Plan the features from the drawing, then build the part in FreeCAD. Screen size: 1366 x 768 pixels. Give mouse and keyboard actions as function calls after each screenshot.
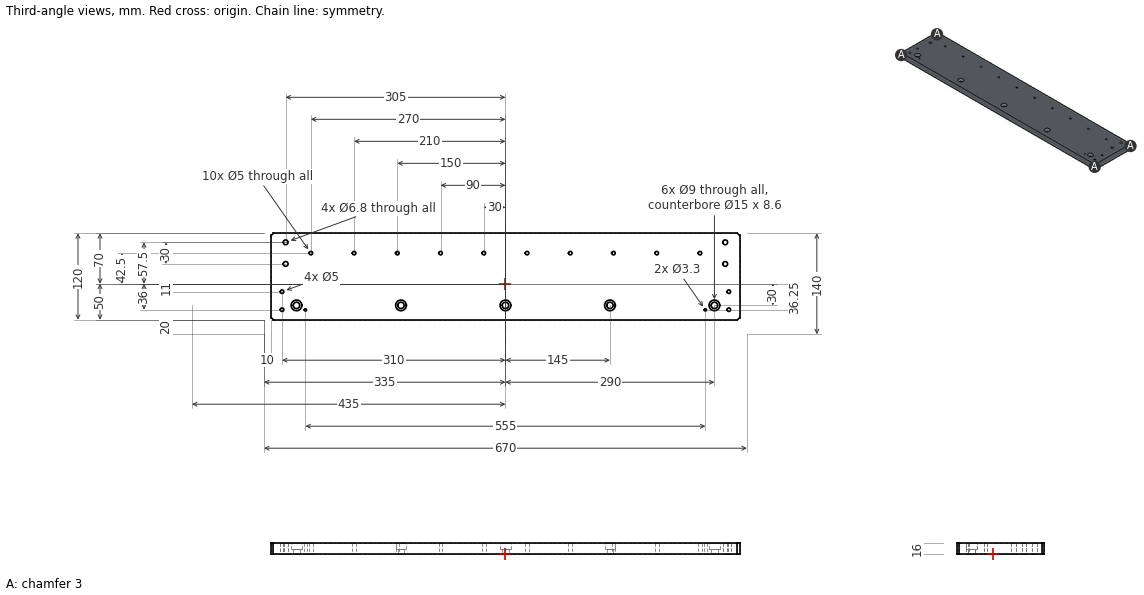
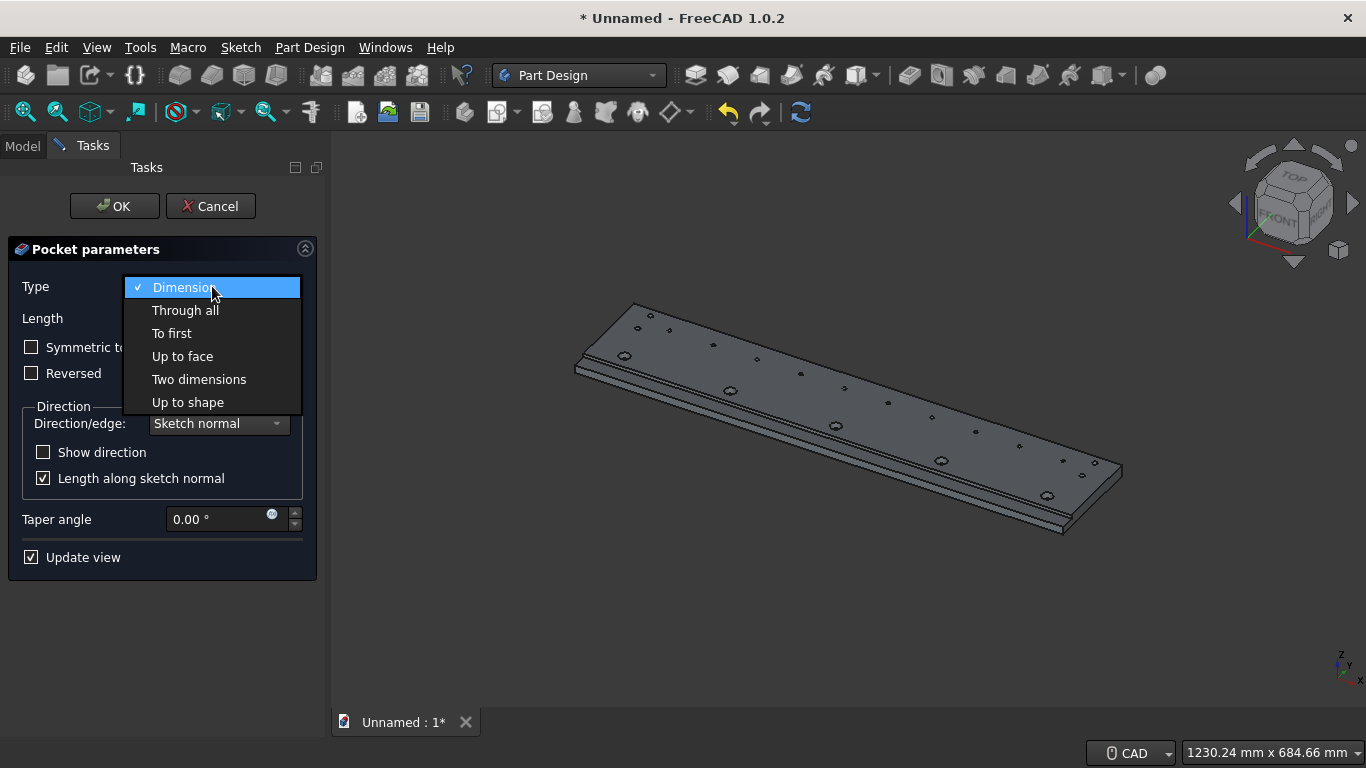
click(212, 310)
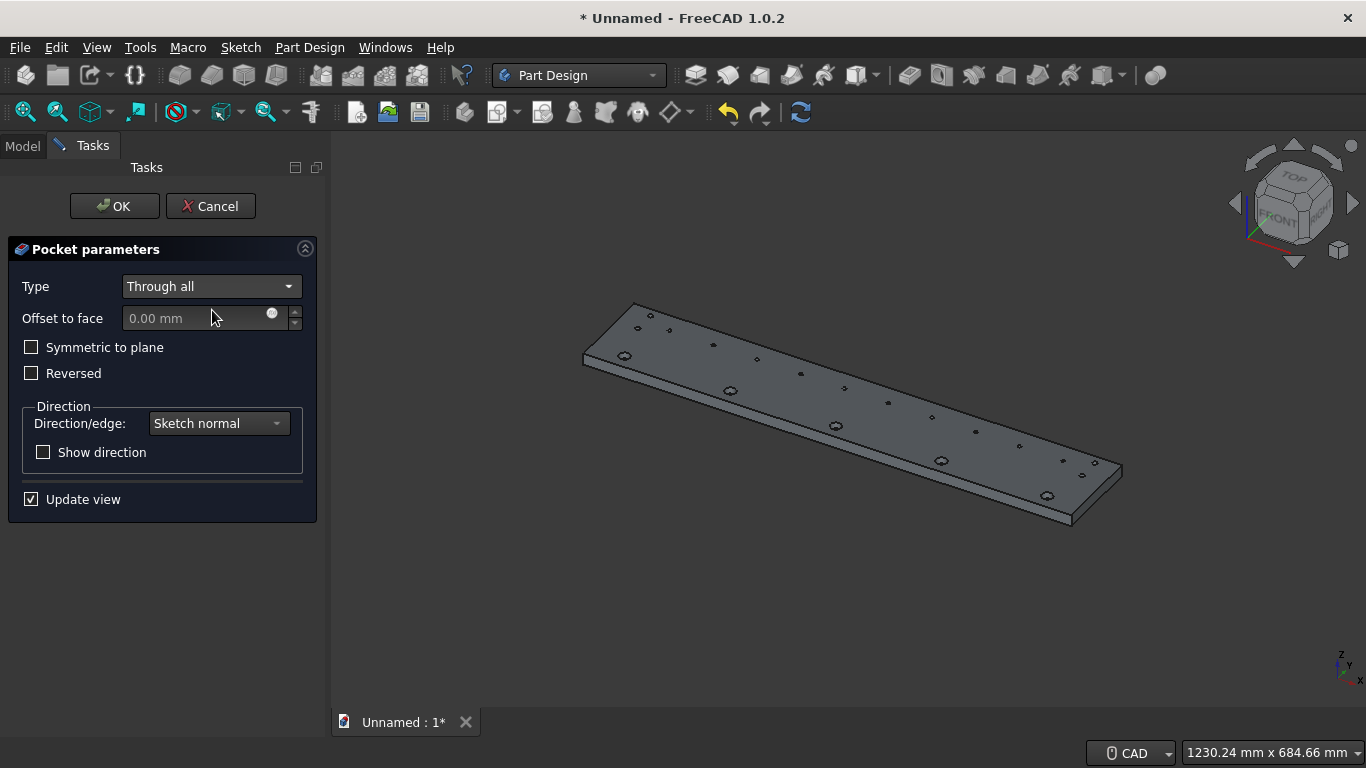
click(115, 206)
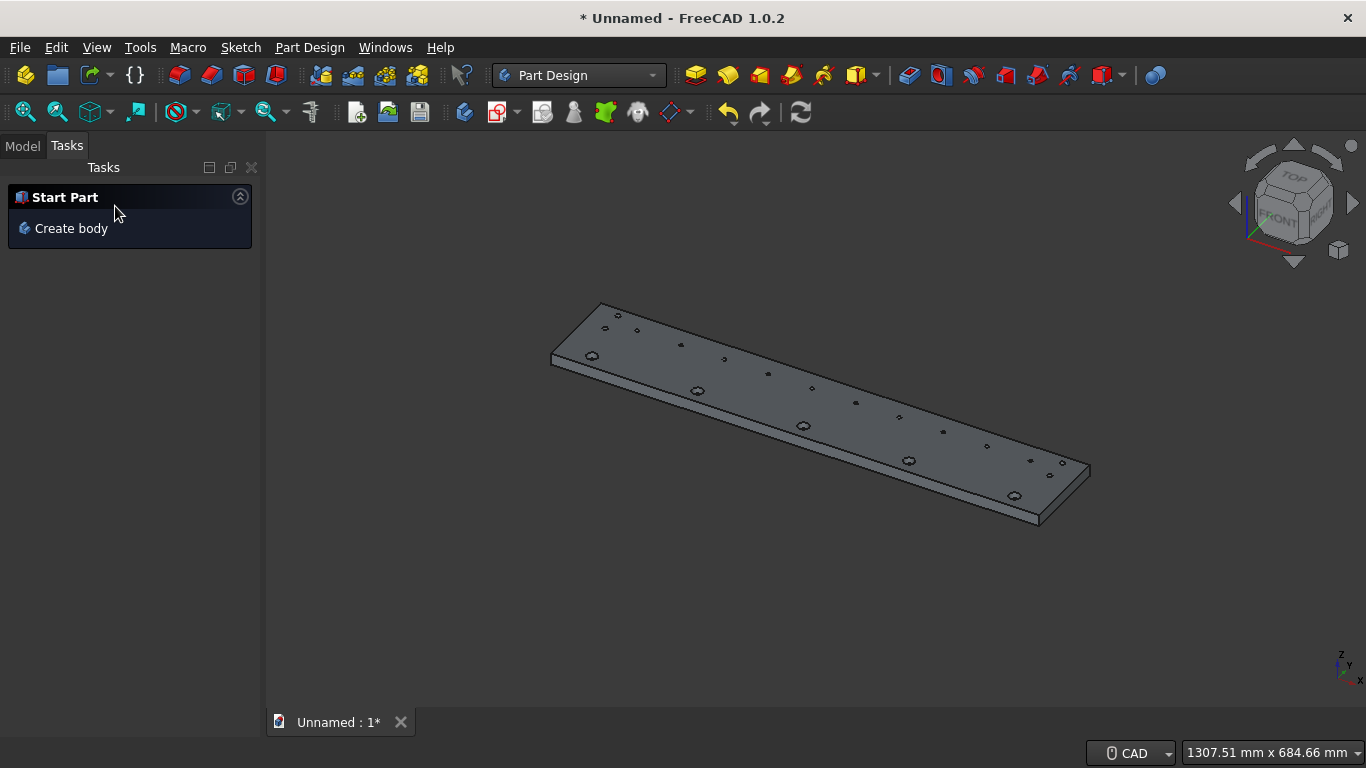
click(952, 462)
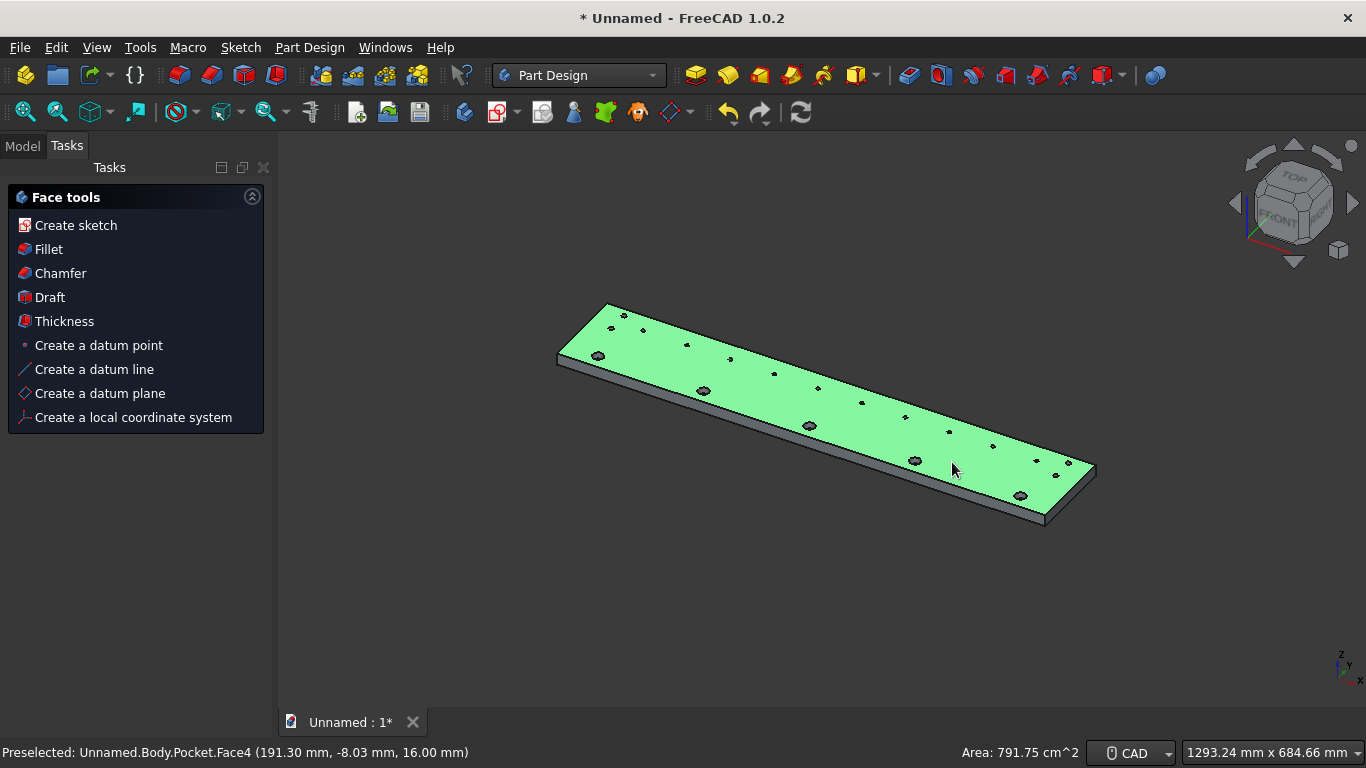
click(498, 112)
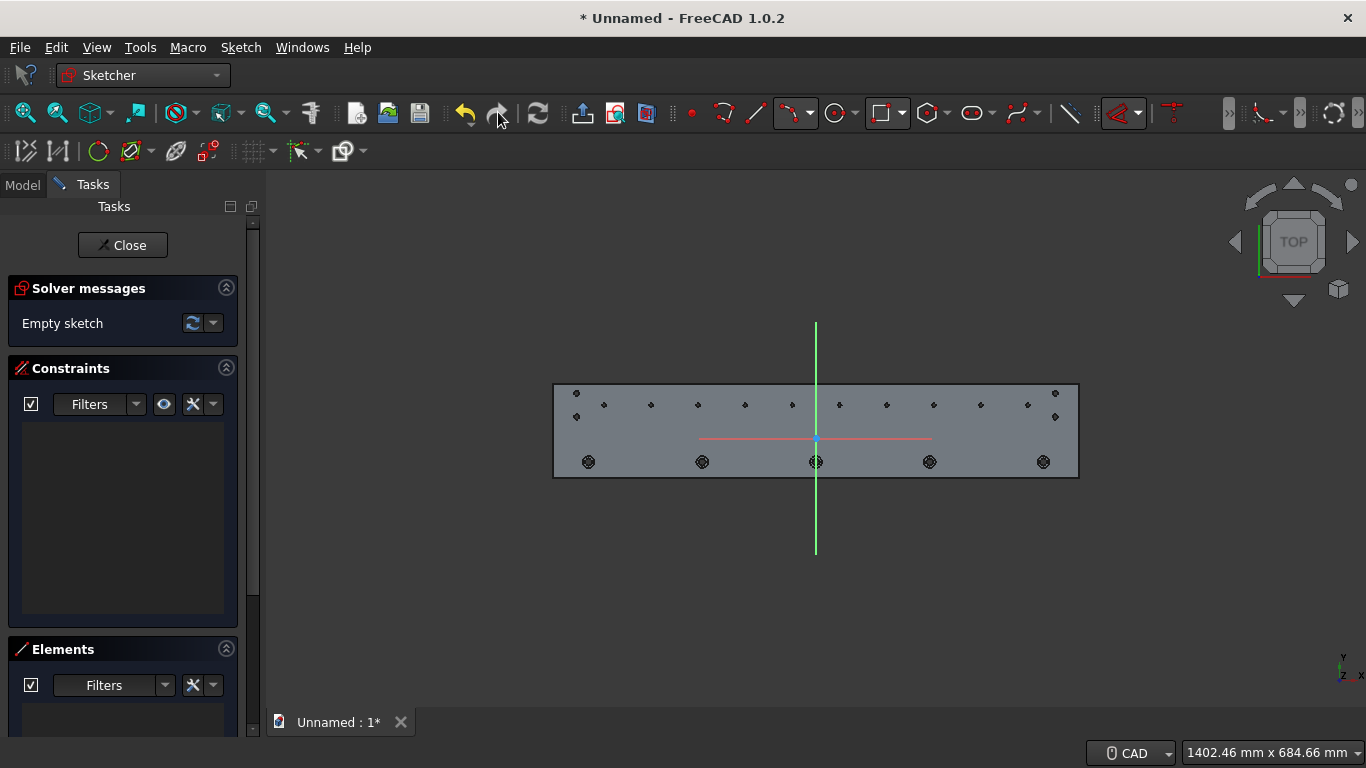
scroll(475, 427, up, 6)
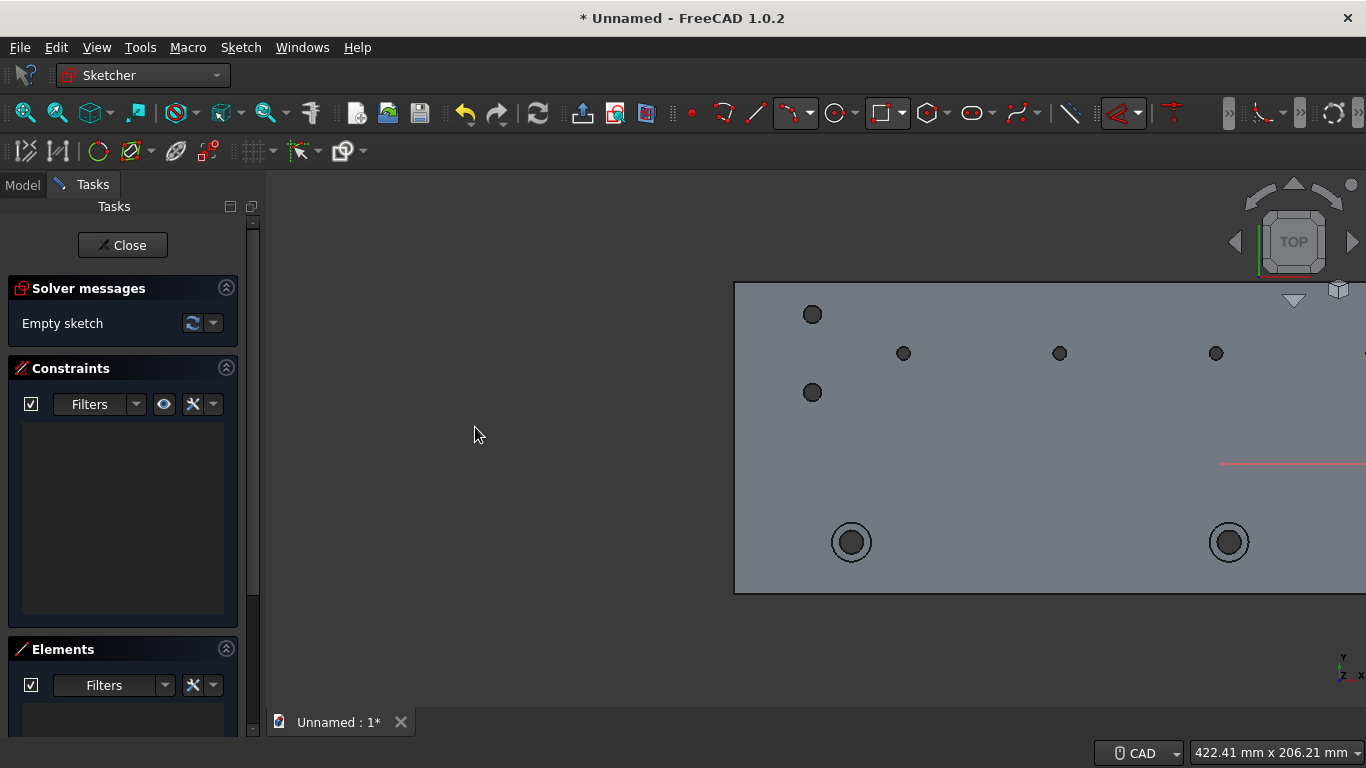
click(882, 114)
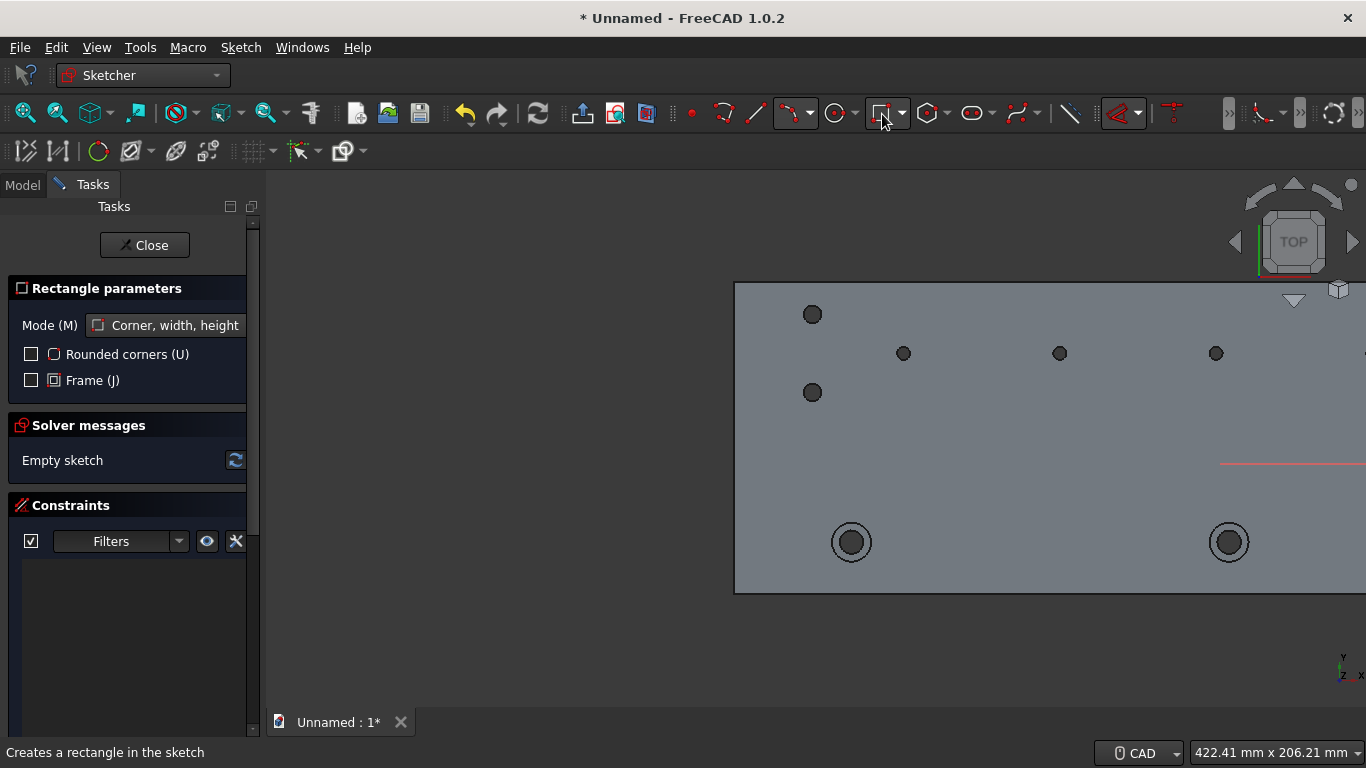
click(734, 282)
click(760, 594)
key(Escape)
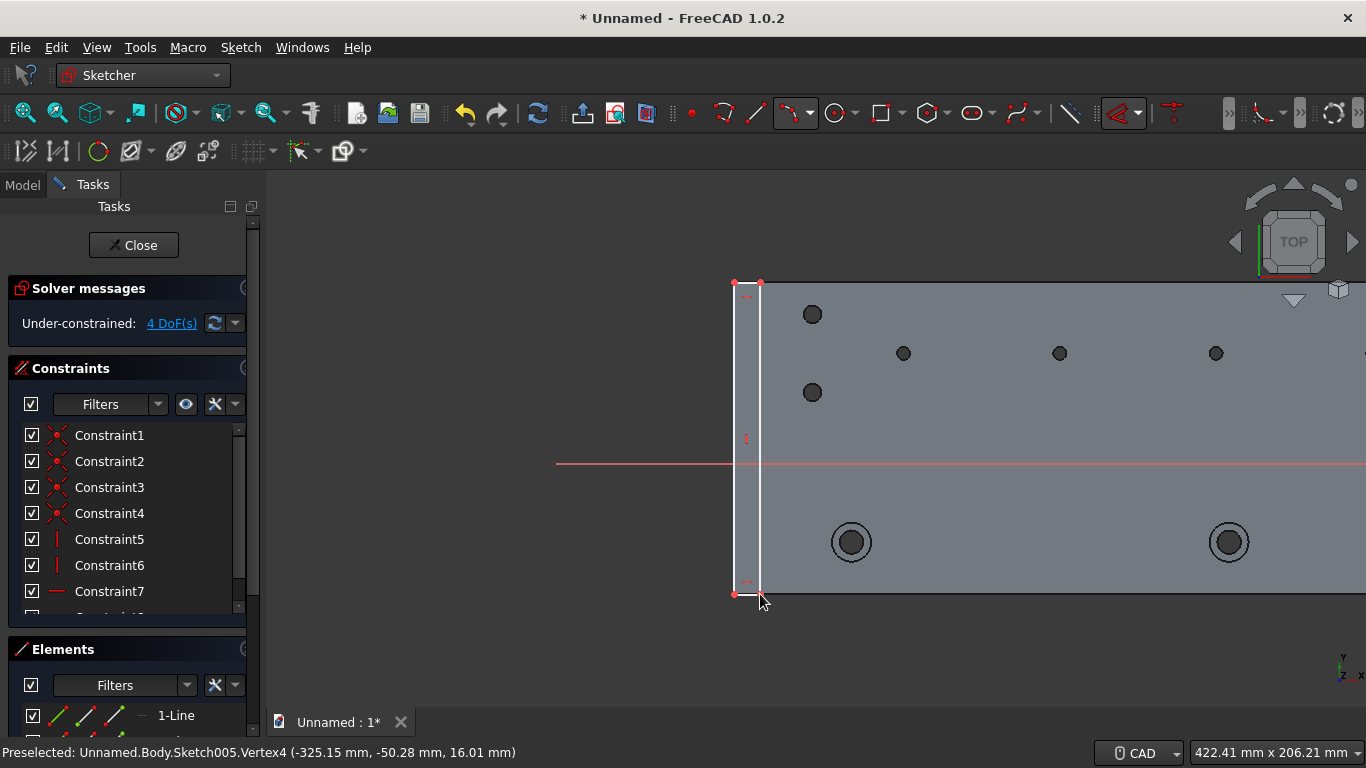
scroll(744, 595, up, 3)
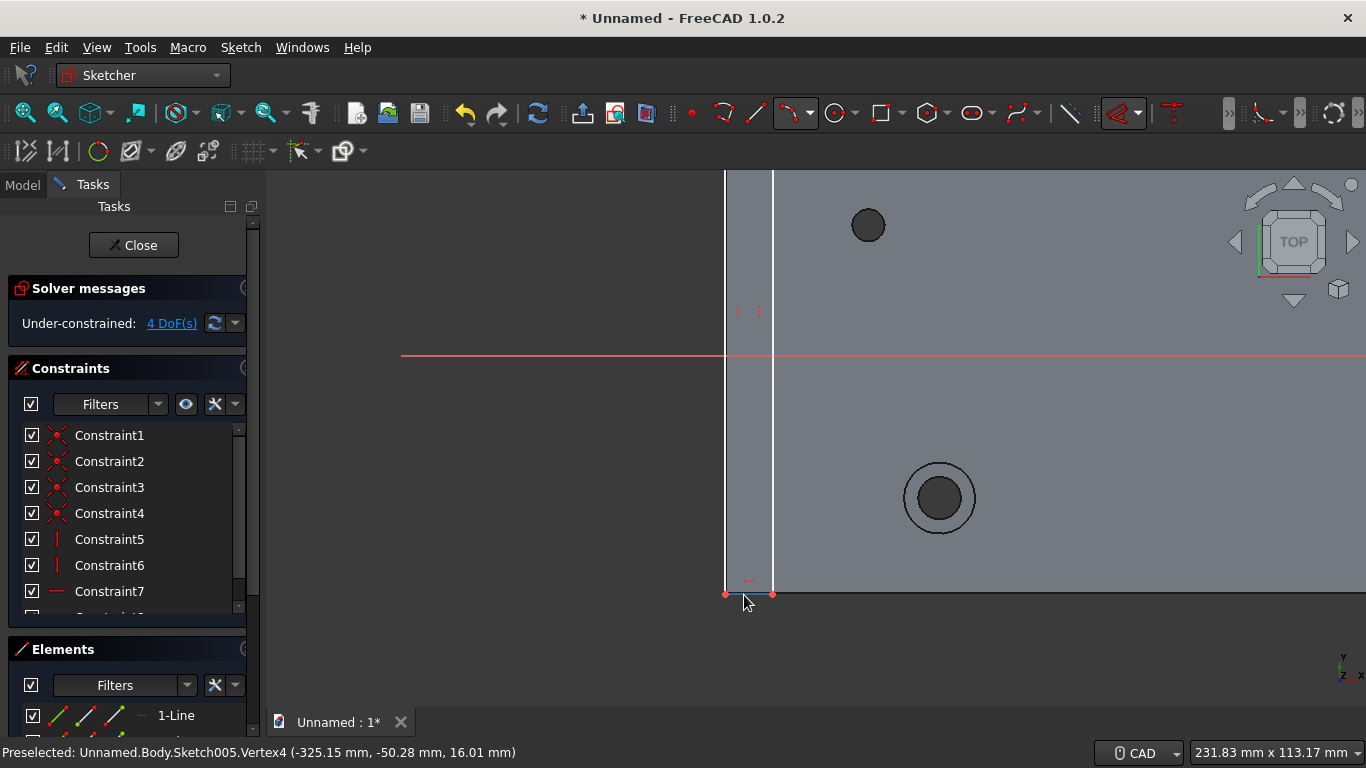
click(744, 594)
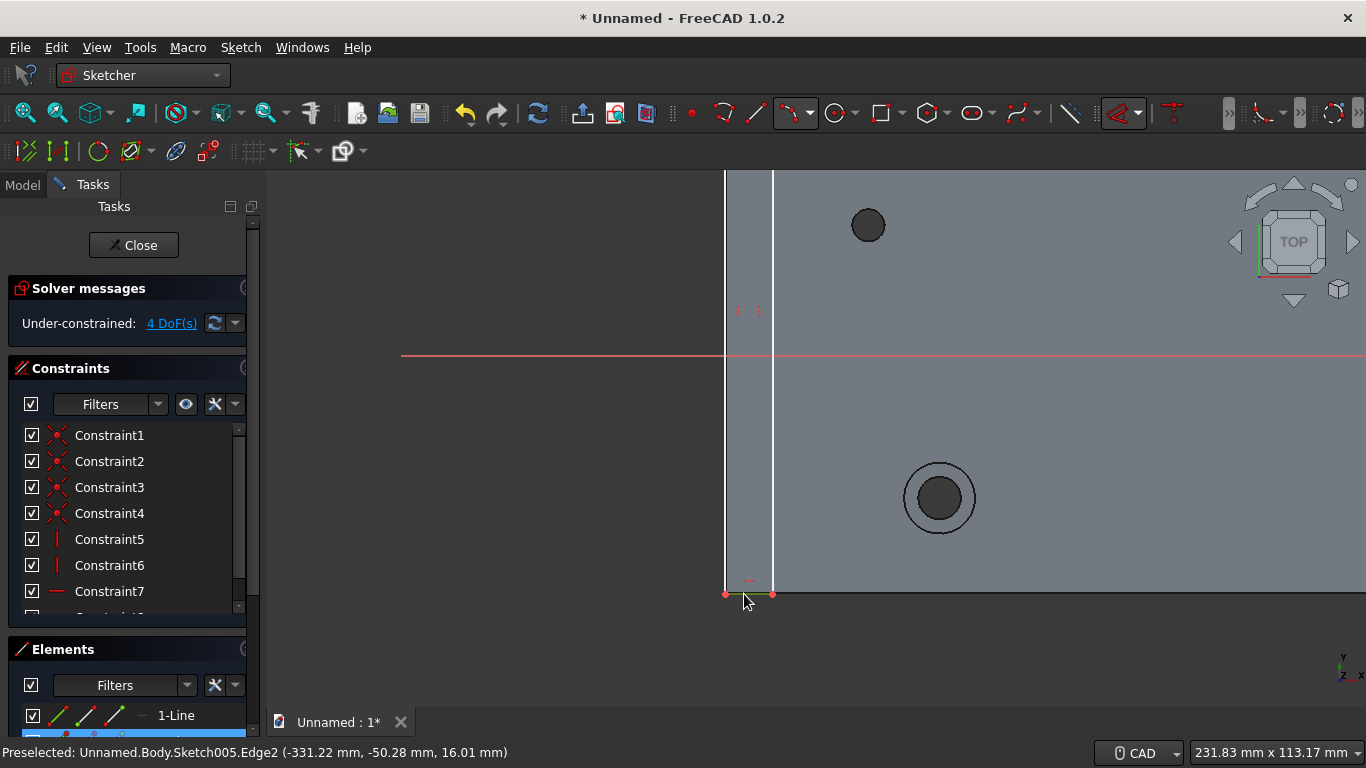
click(1140, 114)